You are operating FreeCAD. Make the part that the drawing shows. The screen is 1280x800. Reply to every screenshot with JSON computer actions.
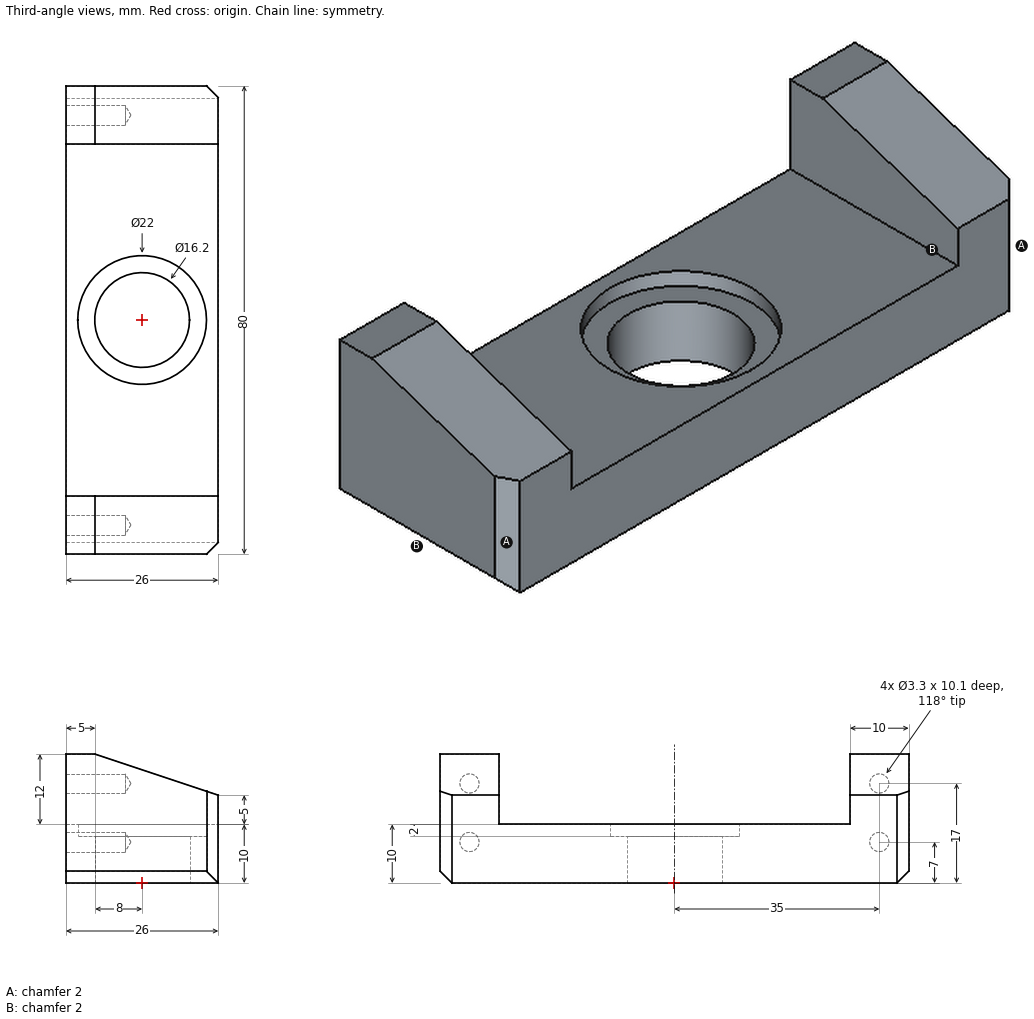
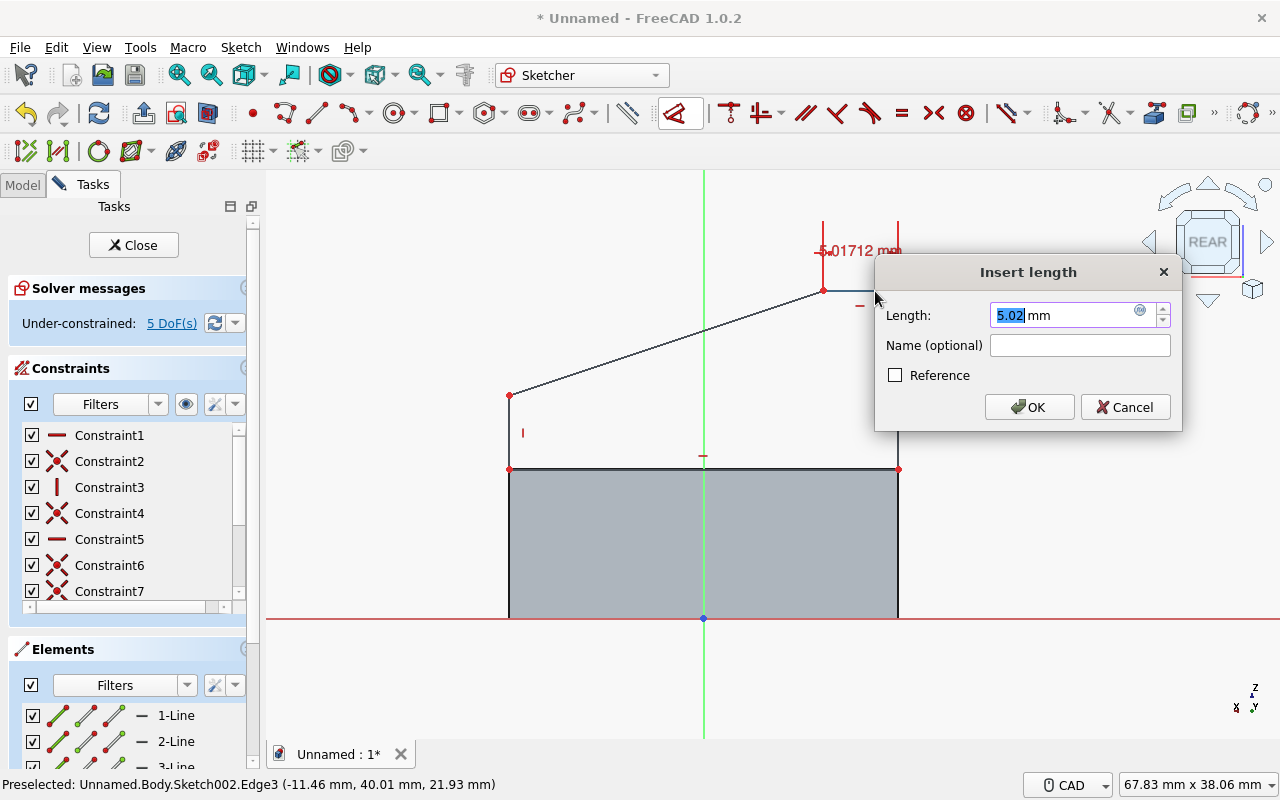
{"action": "type", "text": "5"}
{"action": "key", "text": "Return"}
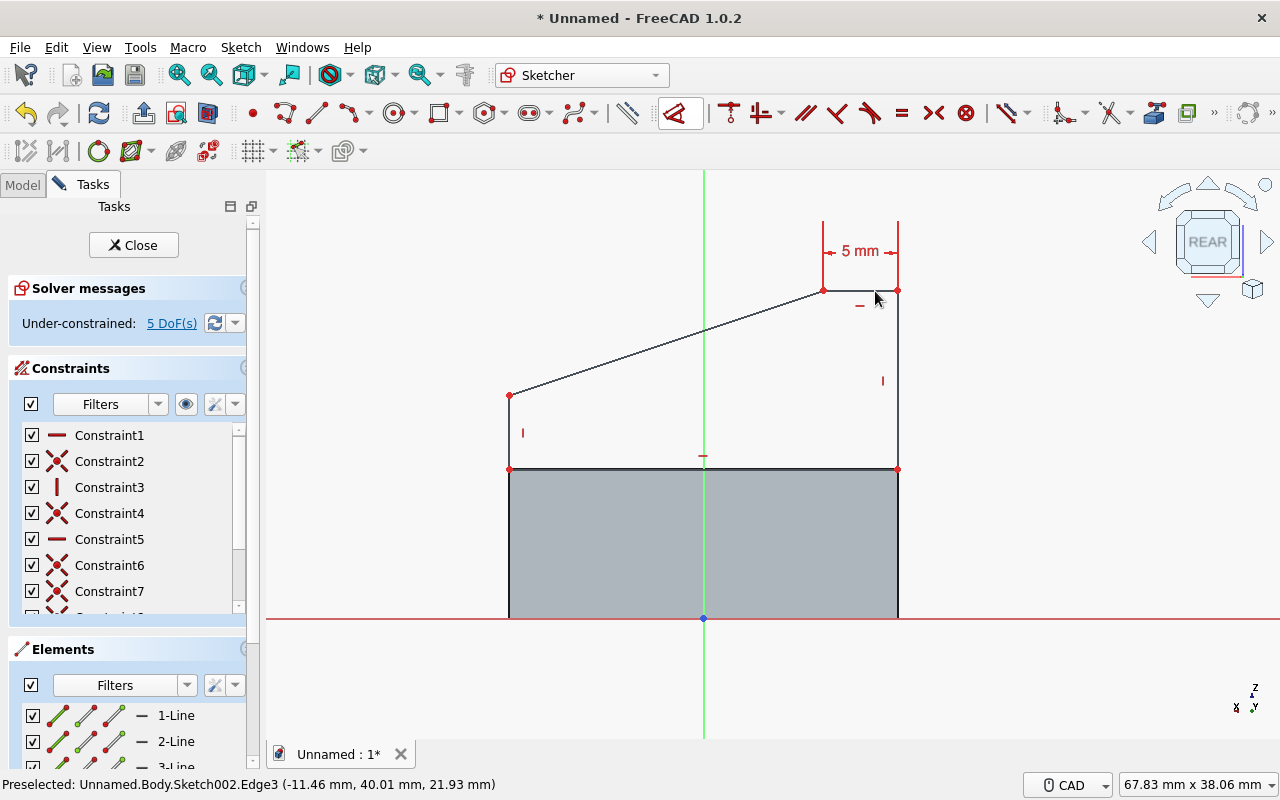
{"action": "left_click", "coordinate": [509, 418]}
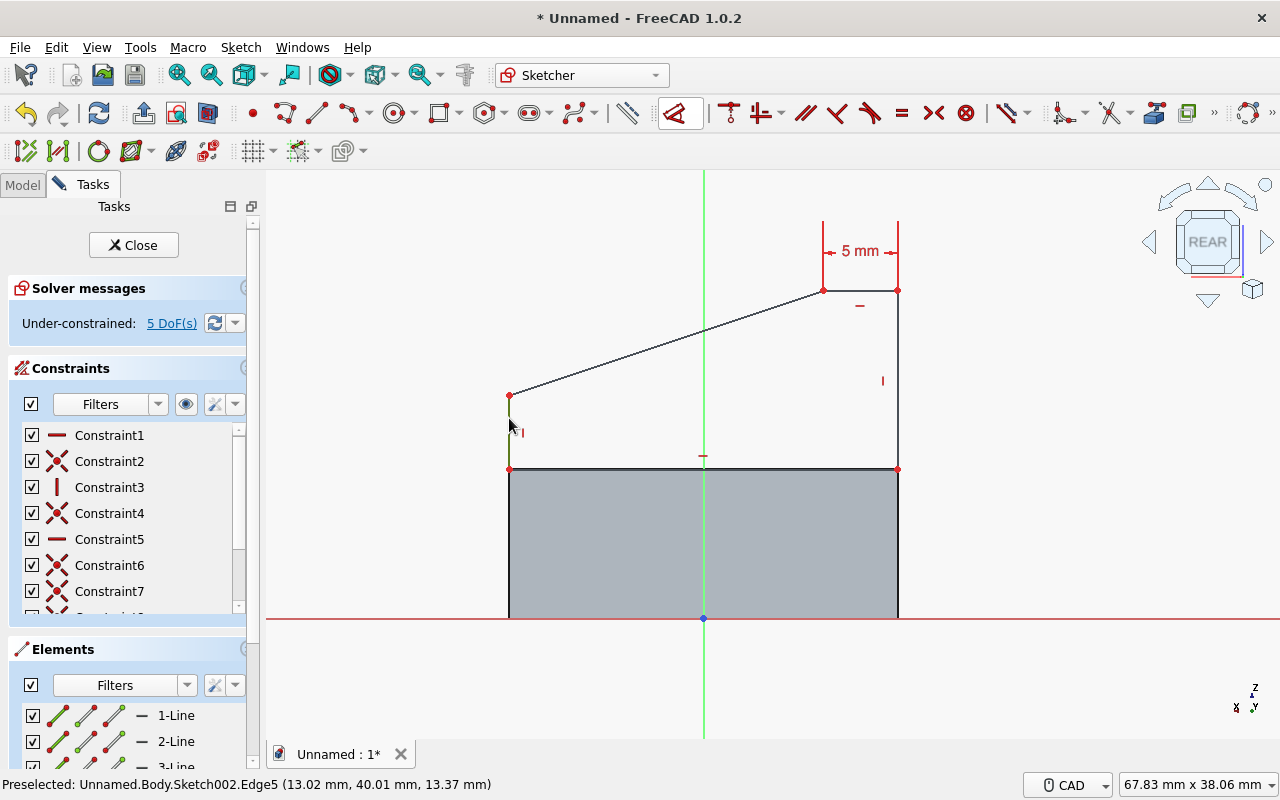
{"action": "key", "text": "i"}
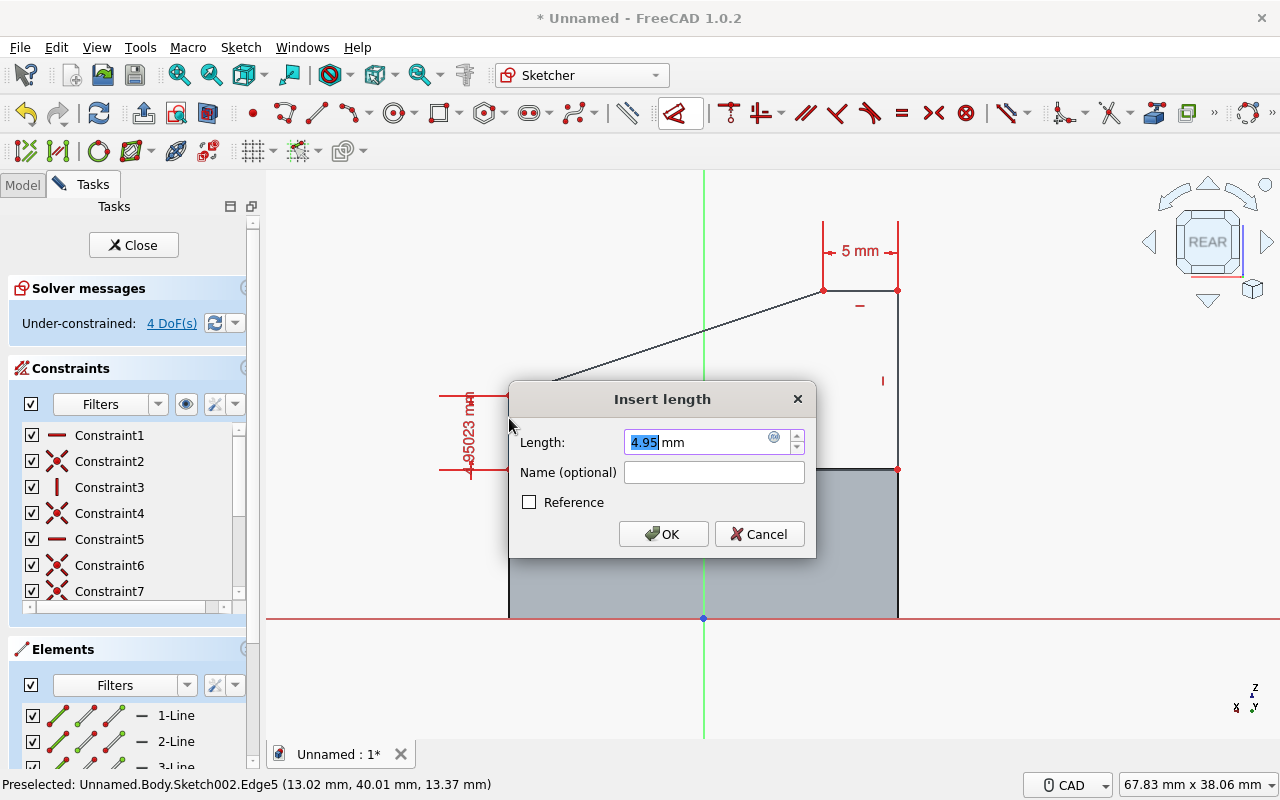
{"action": "type", "text": "5"}
{"action": "key", "text": "Return"}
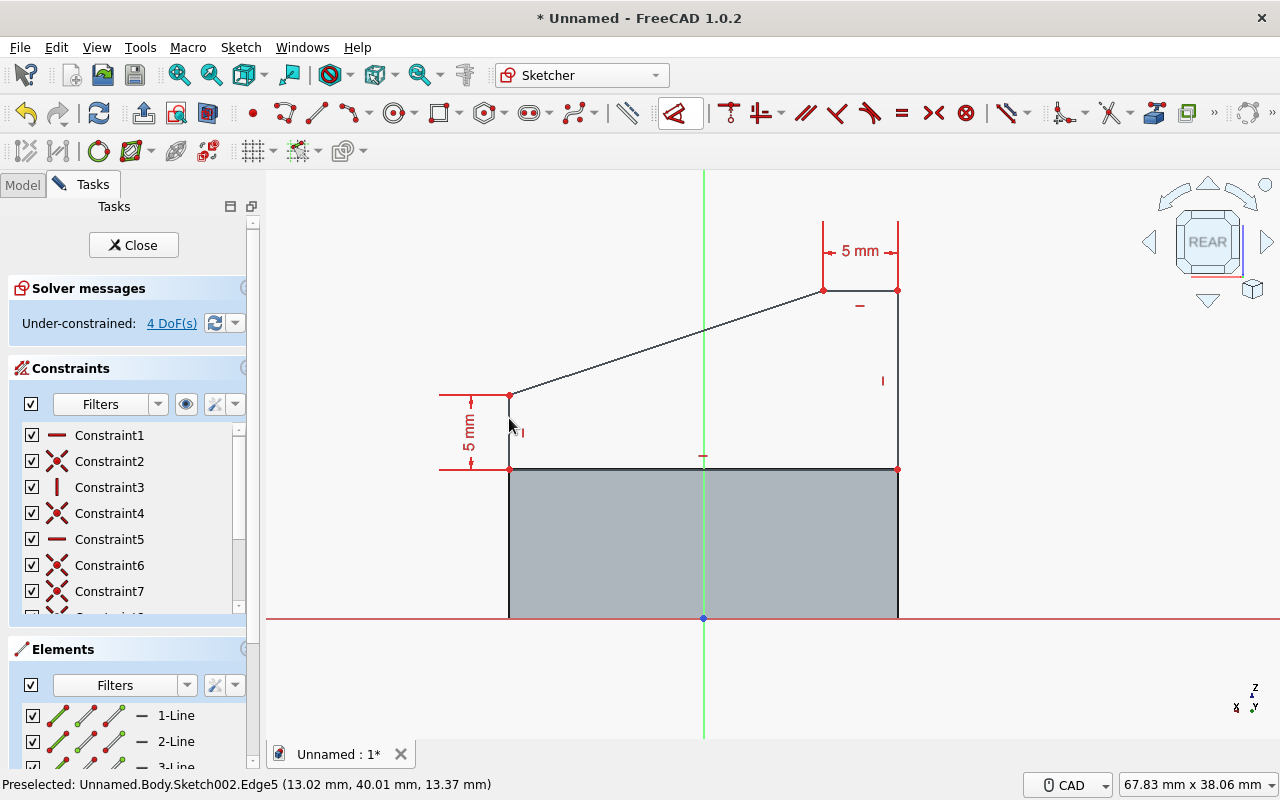
{"action": "left_click", "coordinate": [626, 470]}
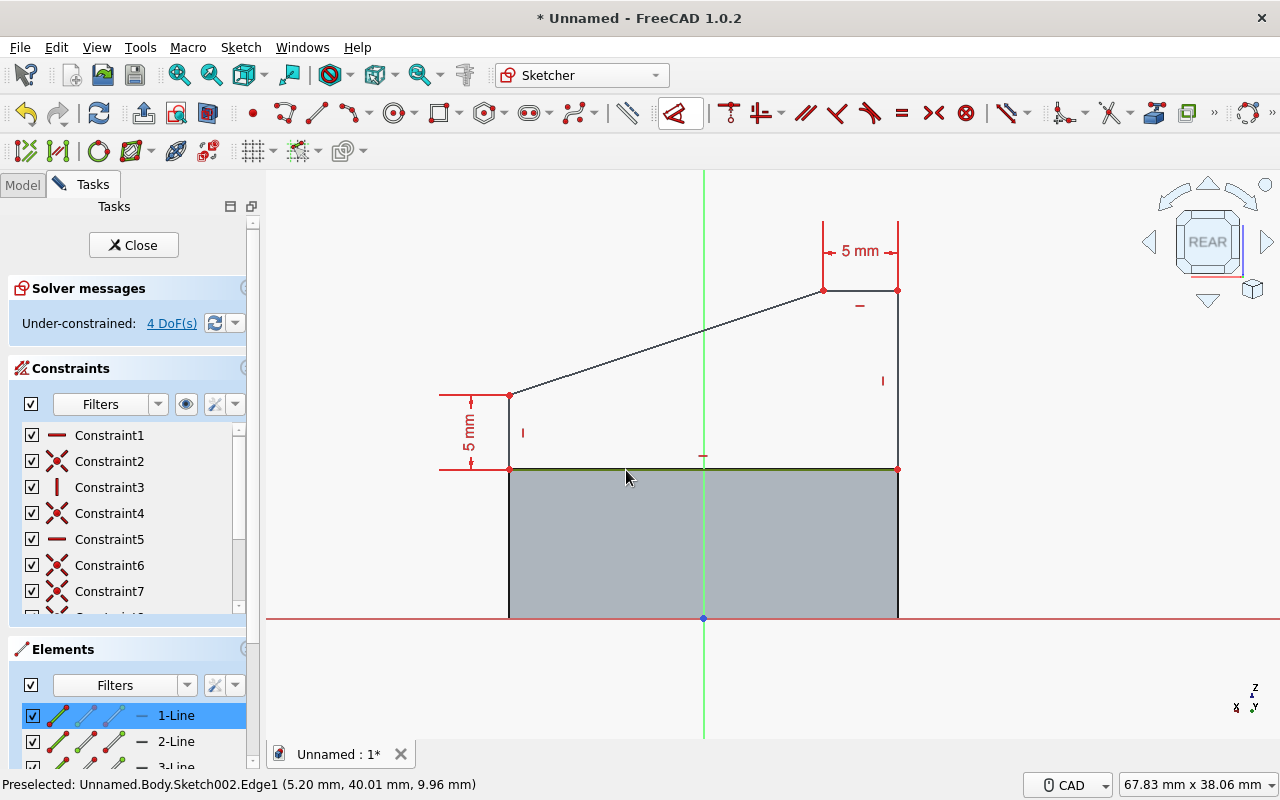
{"action": "left_click", "coordinate": [698, 114]}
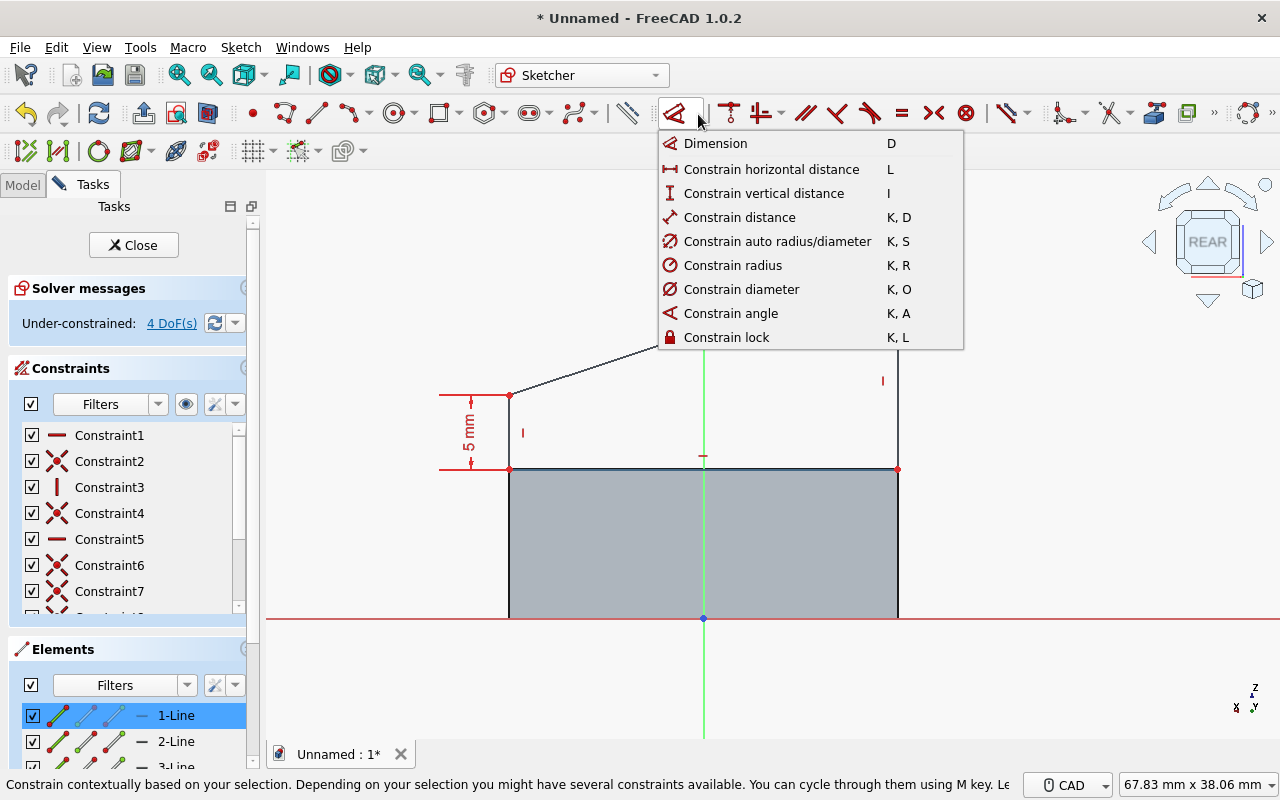
{"action": "left_click", "coordinate": [811, 169]}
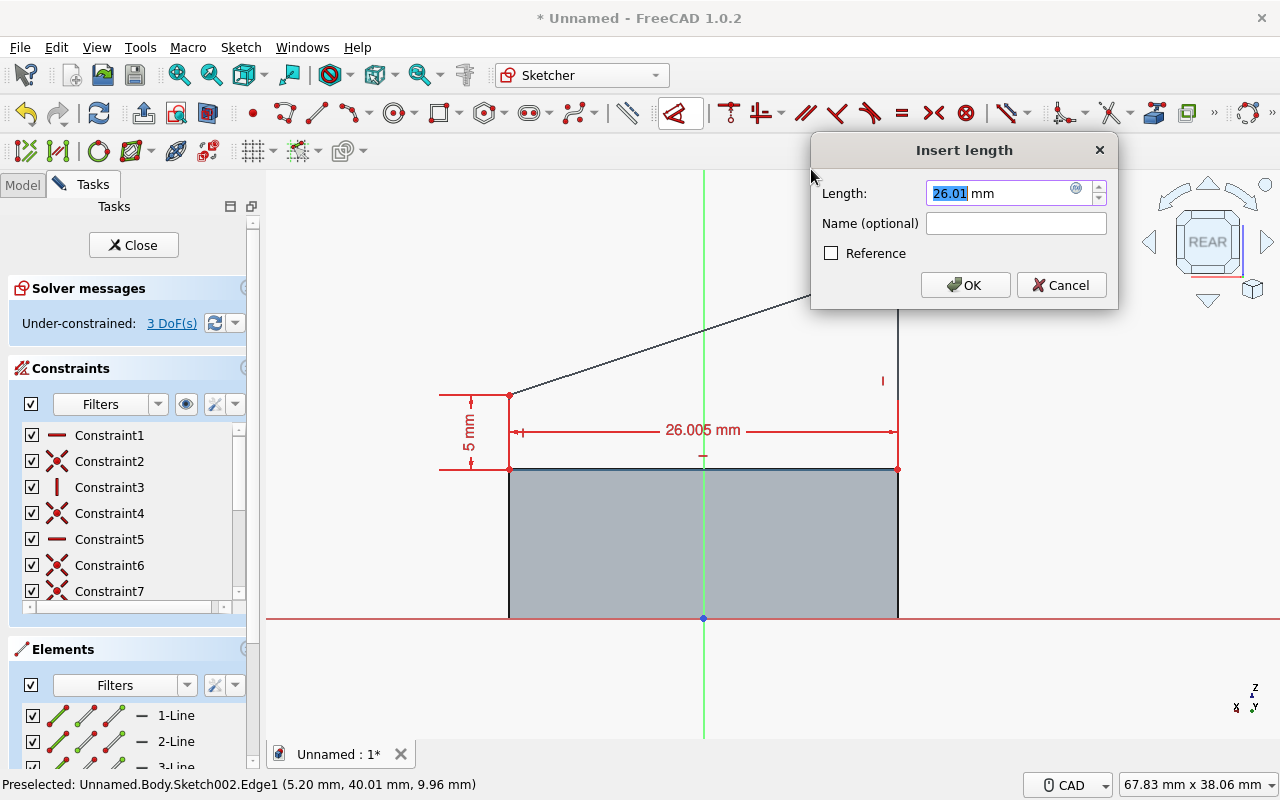
{"action": "type", "text": "26"}
{"action": "key", "text": "Return"}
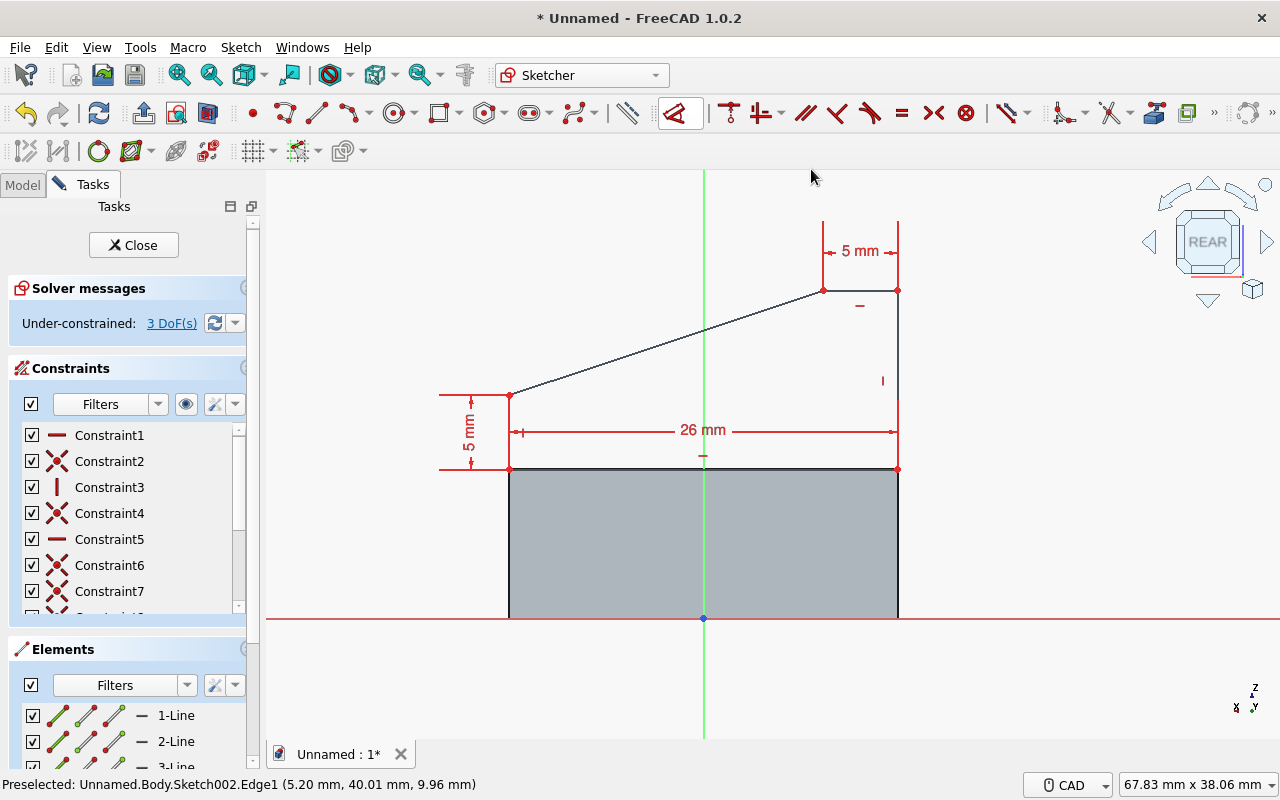
{"action": "left_click", "coordinate": [898, 416]}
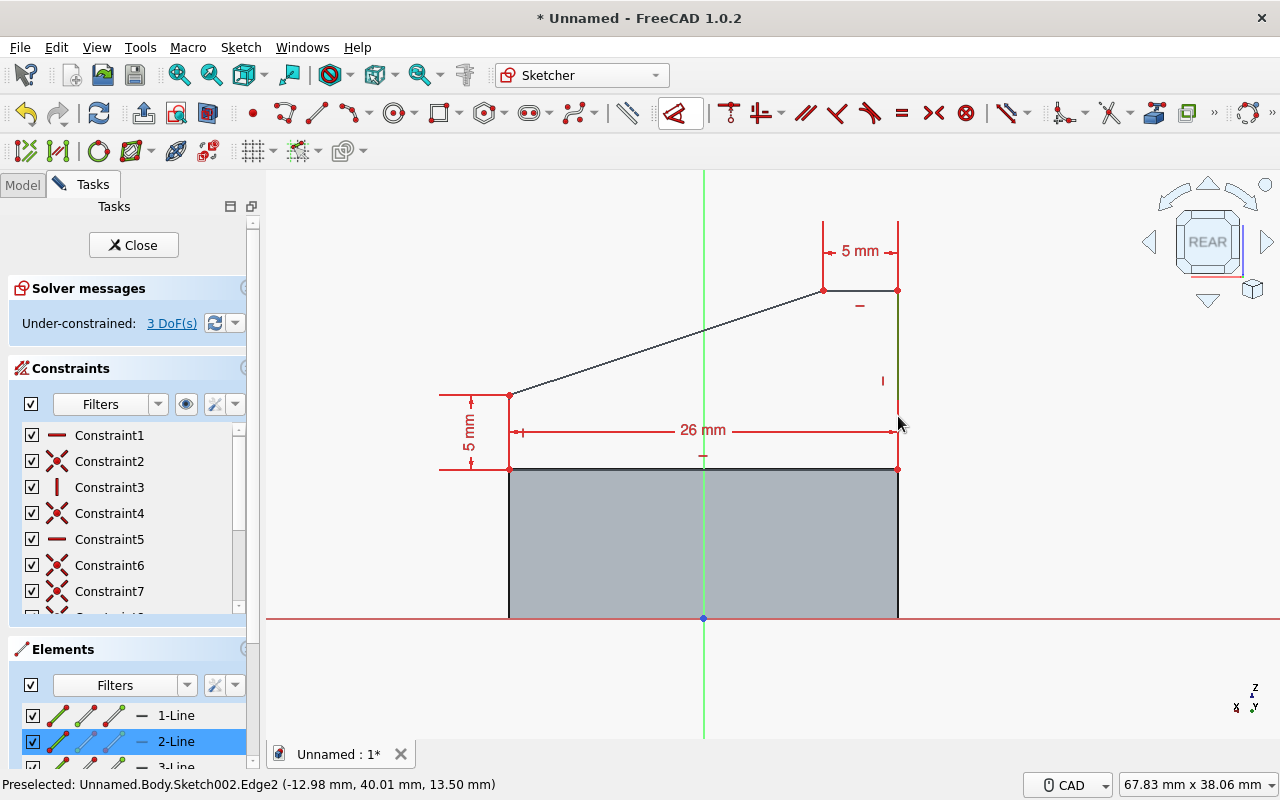
{"action": "left_click", "coordinate": [698, 114]}